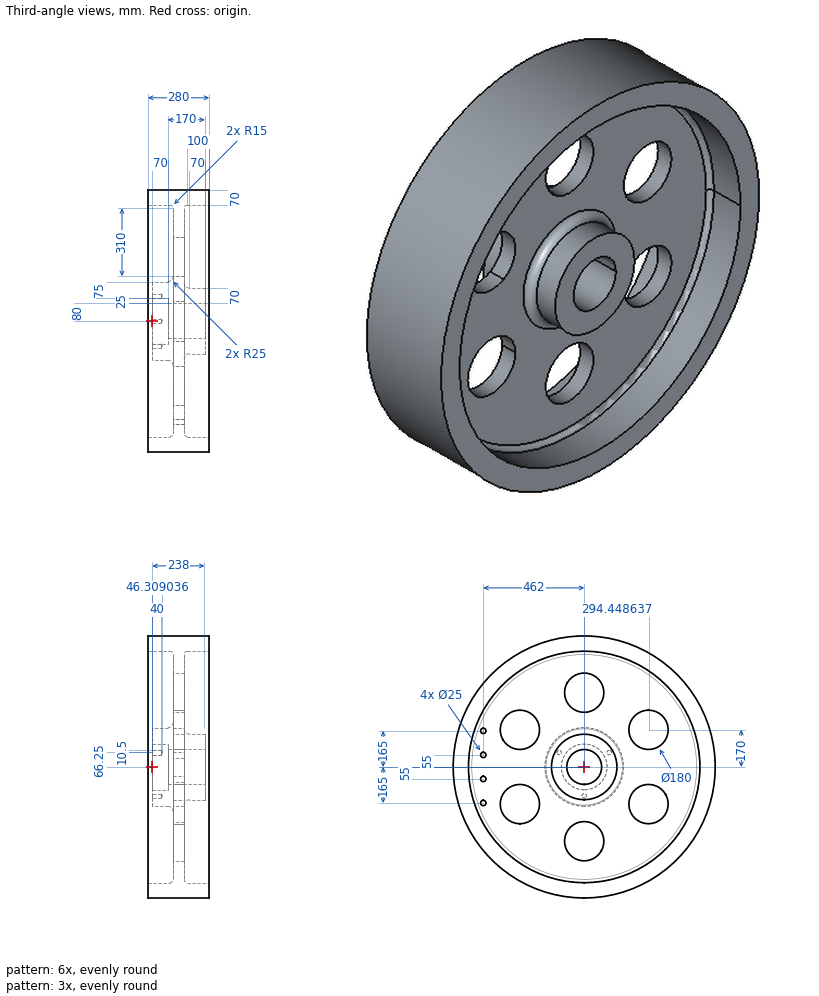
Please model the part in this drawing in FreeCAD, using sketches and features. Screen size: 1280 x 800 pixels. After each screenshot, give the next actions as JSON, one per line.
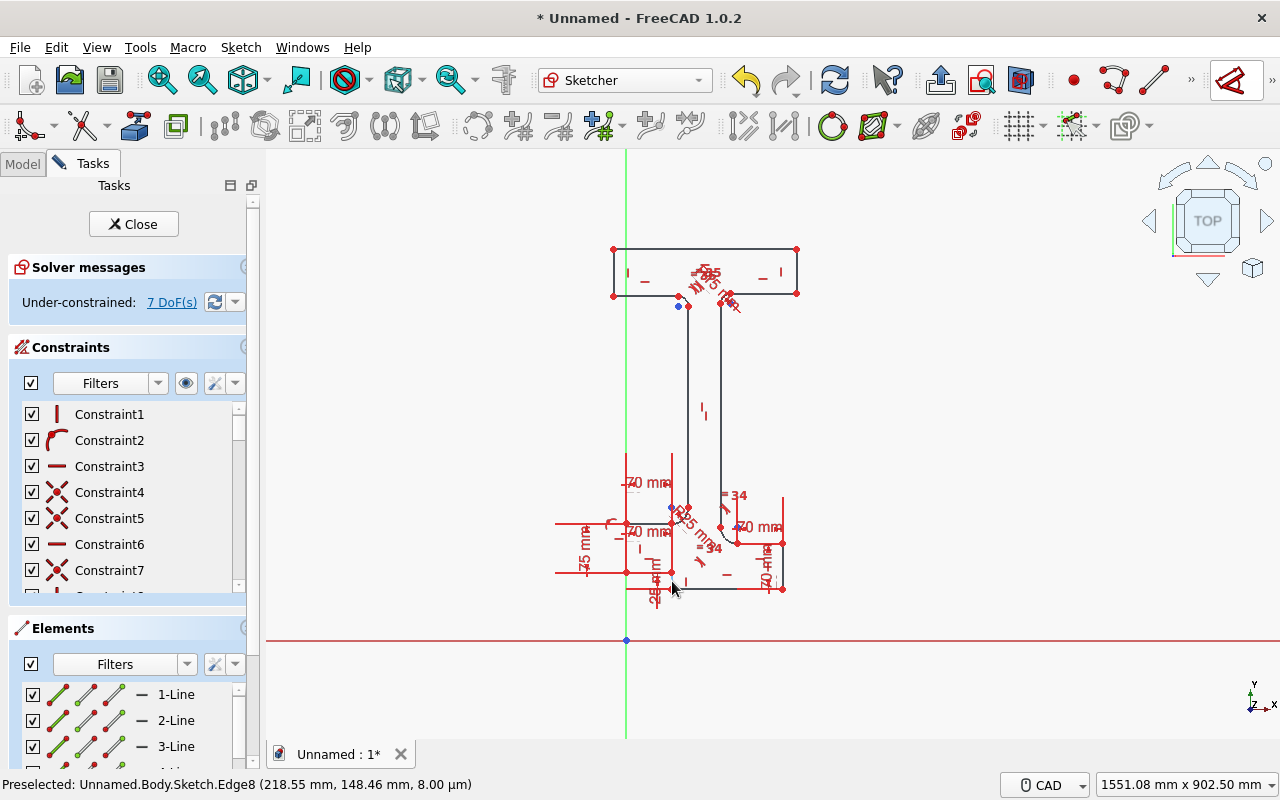
{"action": "left_click", "coordinate": [797, 280]}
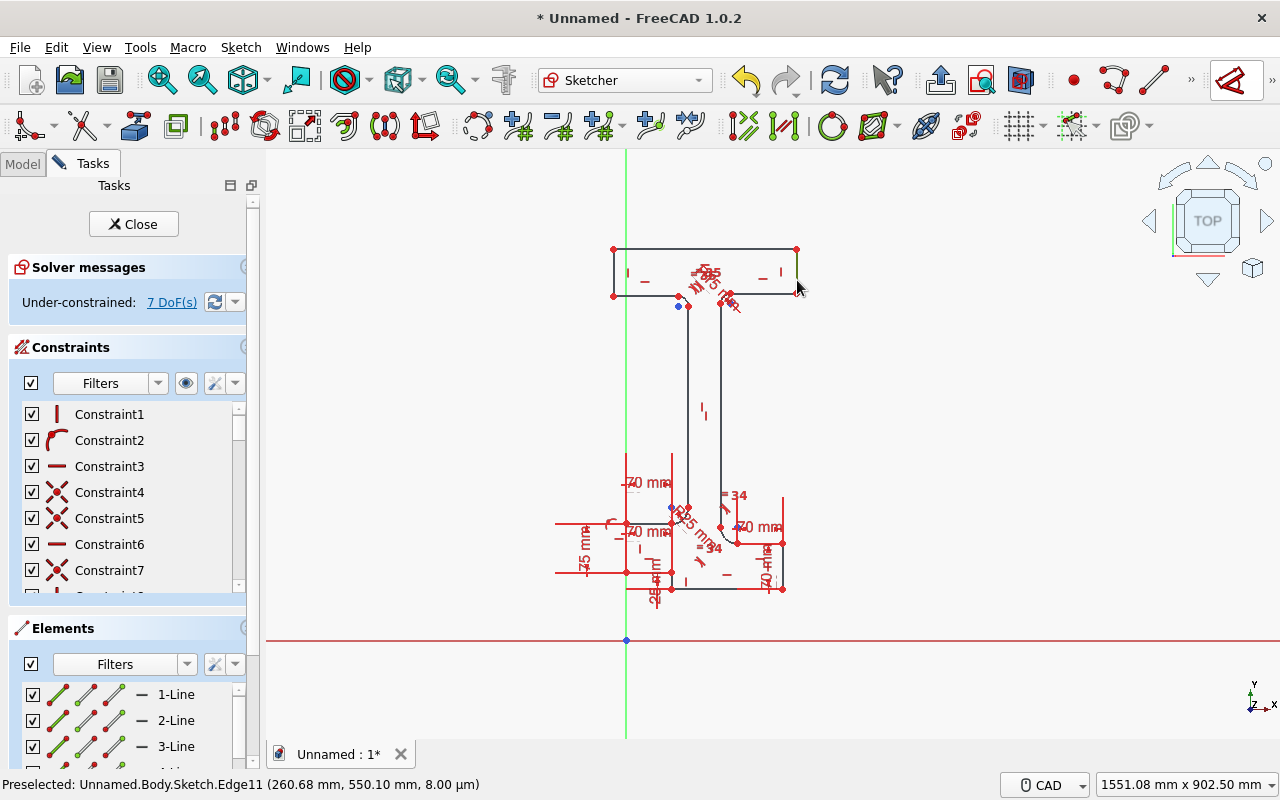
{"action": "left_click", "coordinate": [1258, 80]}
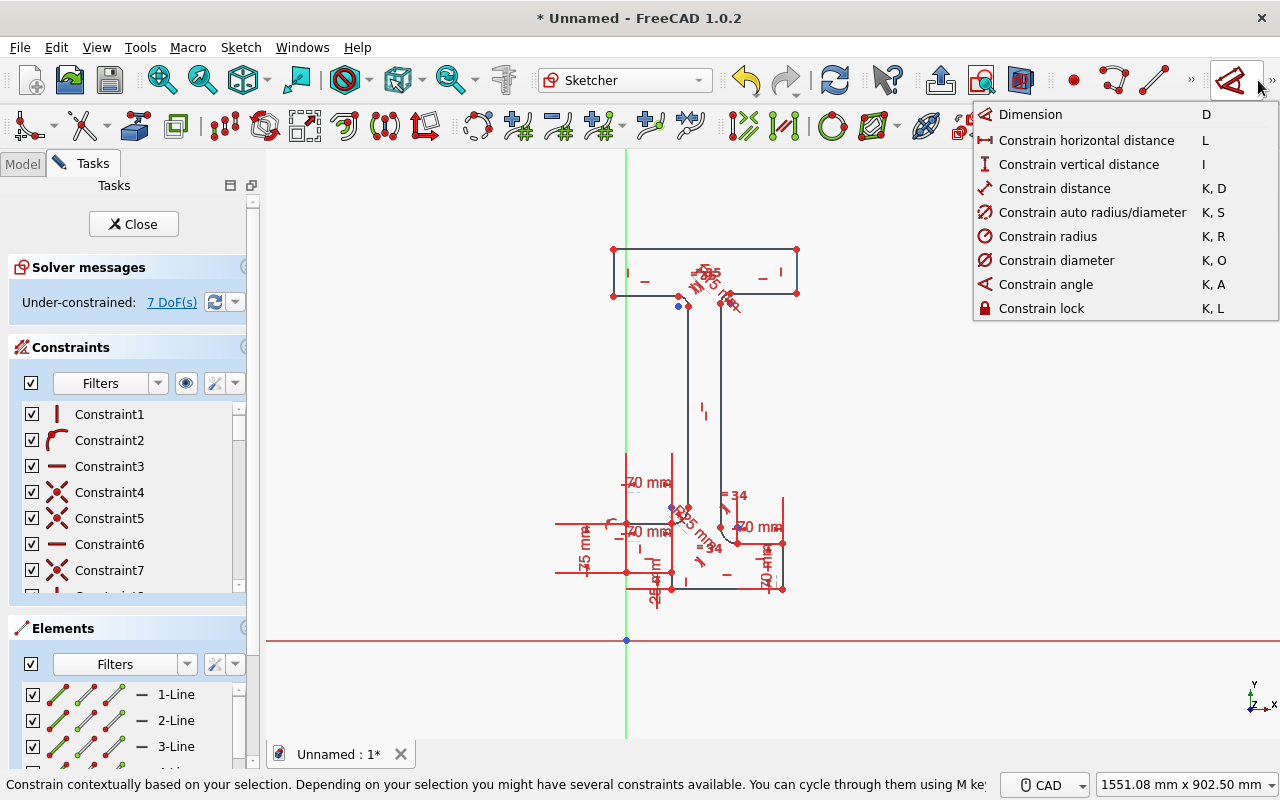
{"action": "left_click", "coordinate": [1126, 164]}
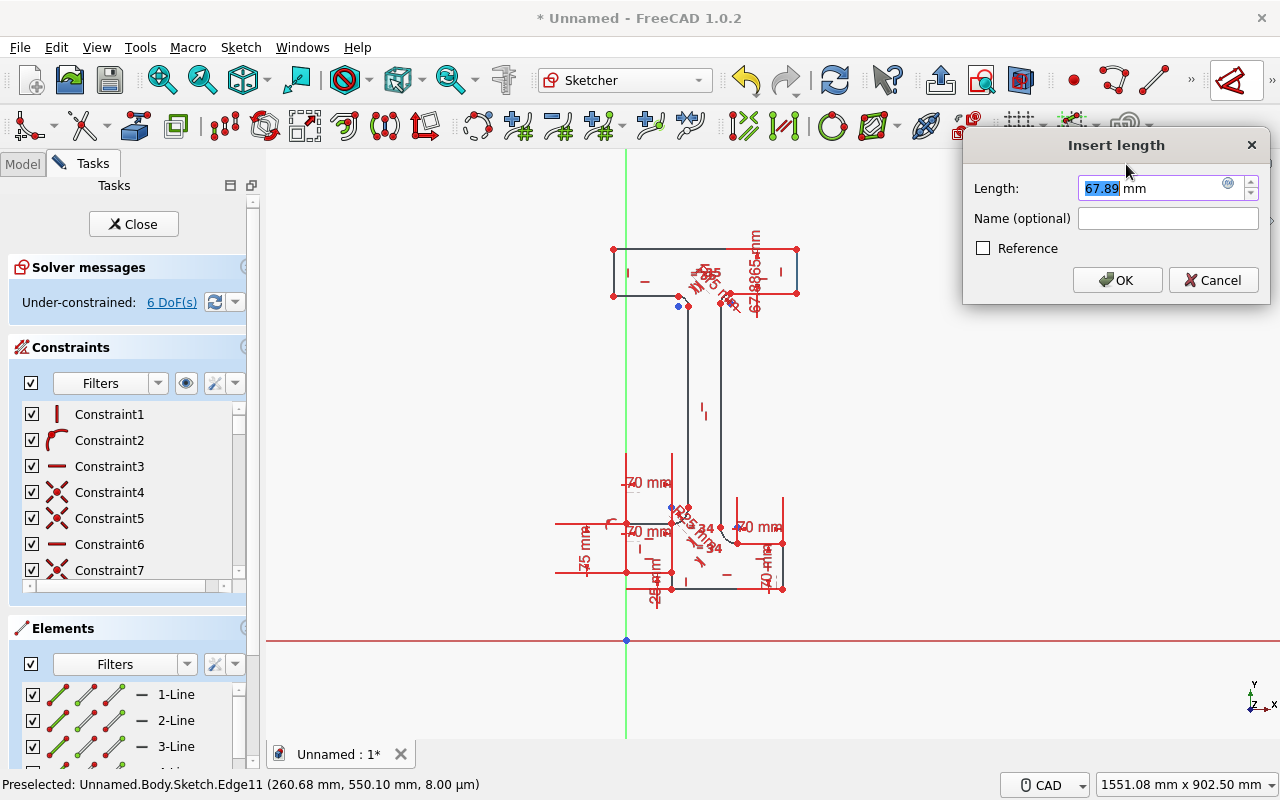
{"action": "type", "text": "70"}
{"action": "key", "text": "Return"}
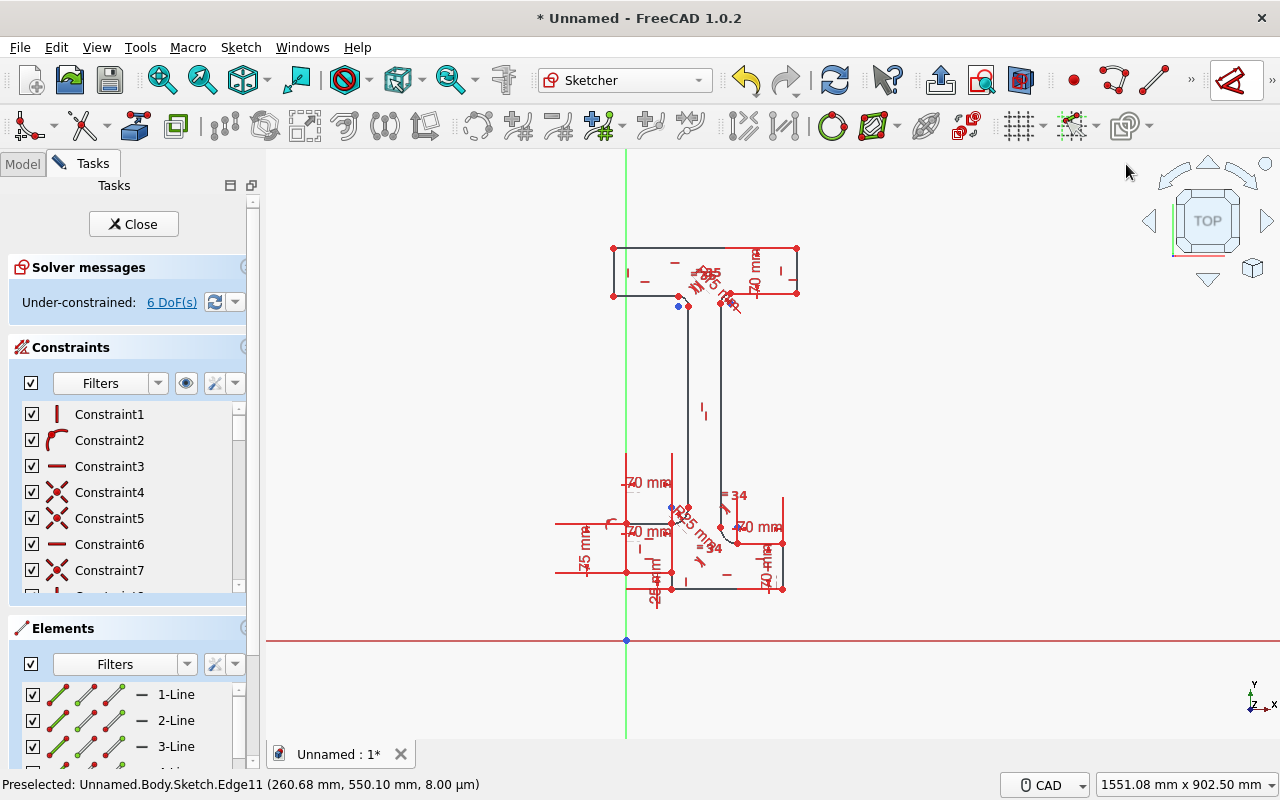
{"action": "left_click", "coordinate": [614, 262]}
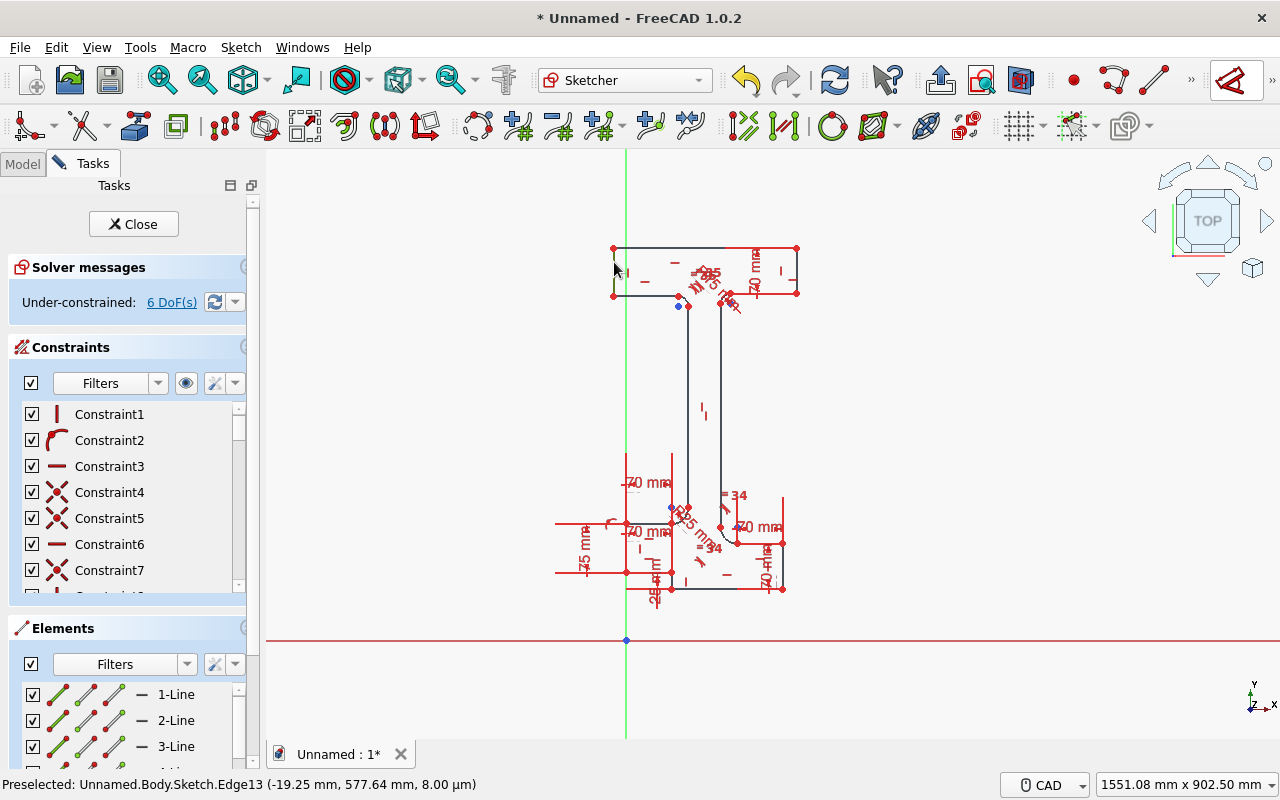
{"action": "key", "text": "i"}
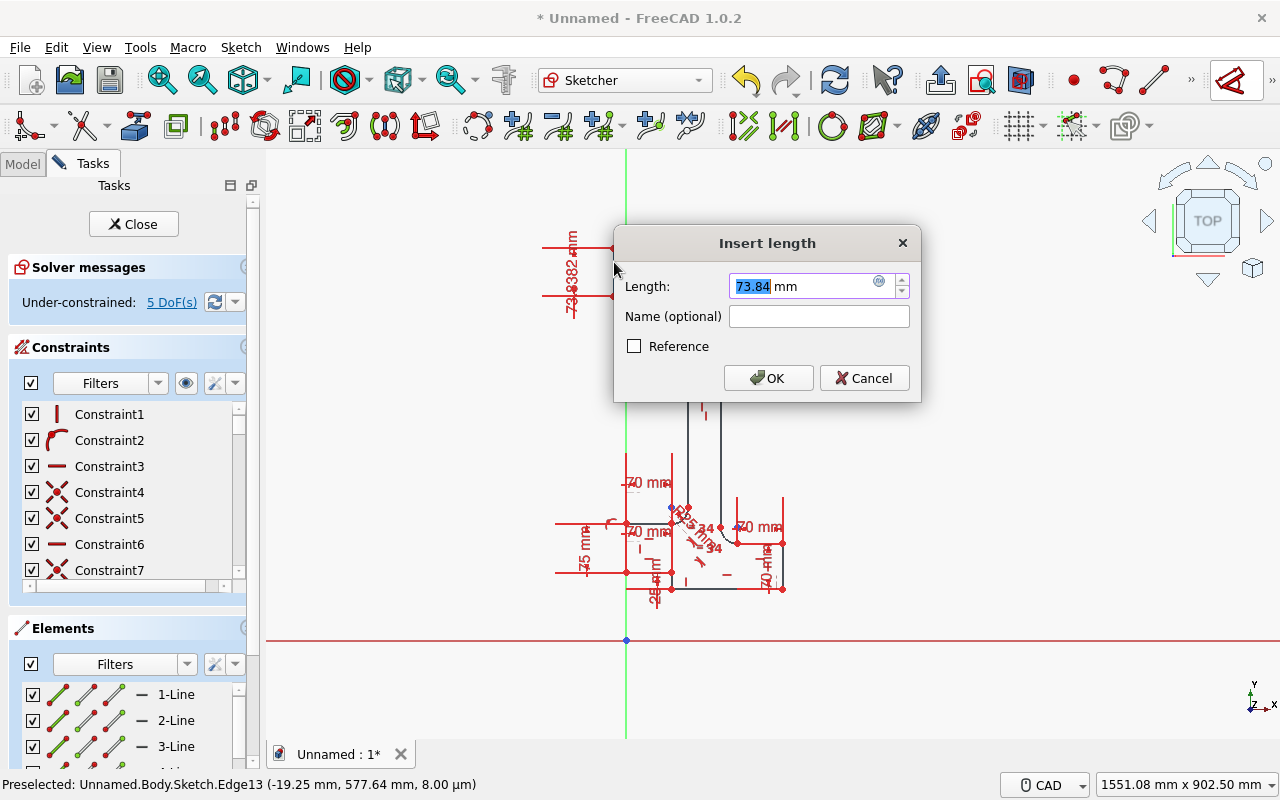
{"action": "type", "text": "70"}
{"action": "key", "text": "Return"}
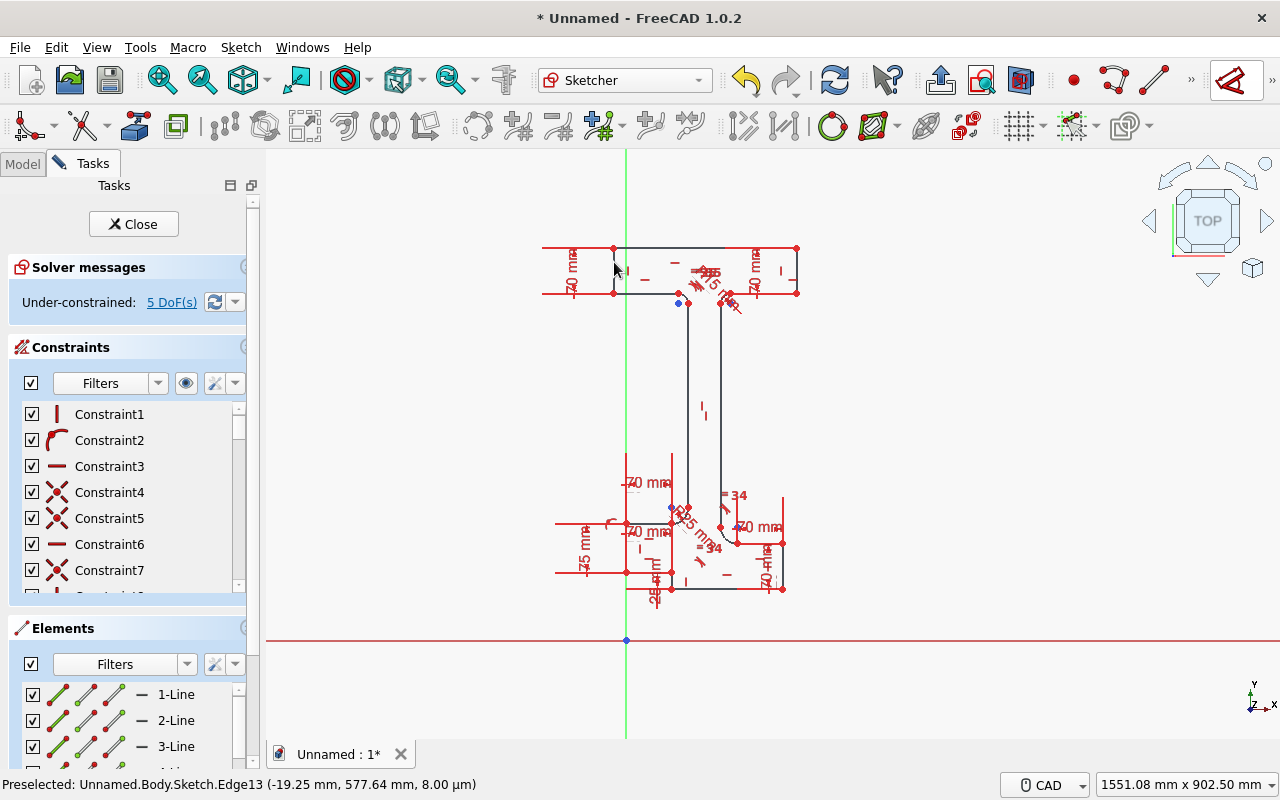
{"action": "left_click", "coordinate": [688, 365]}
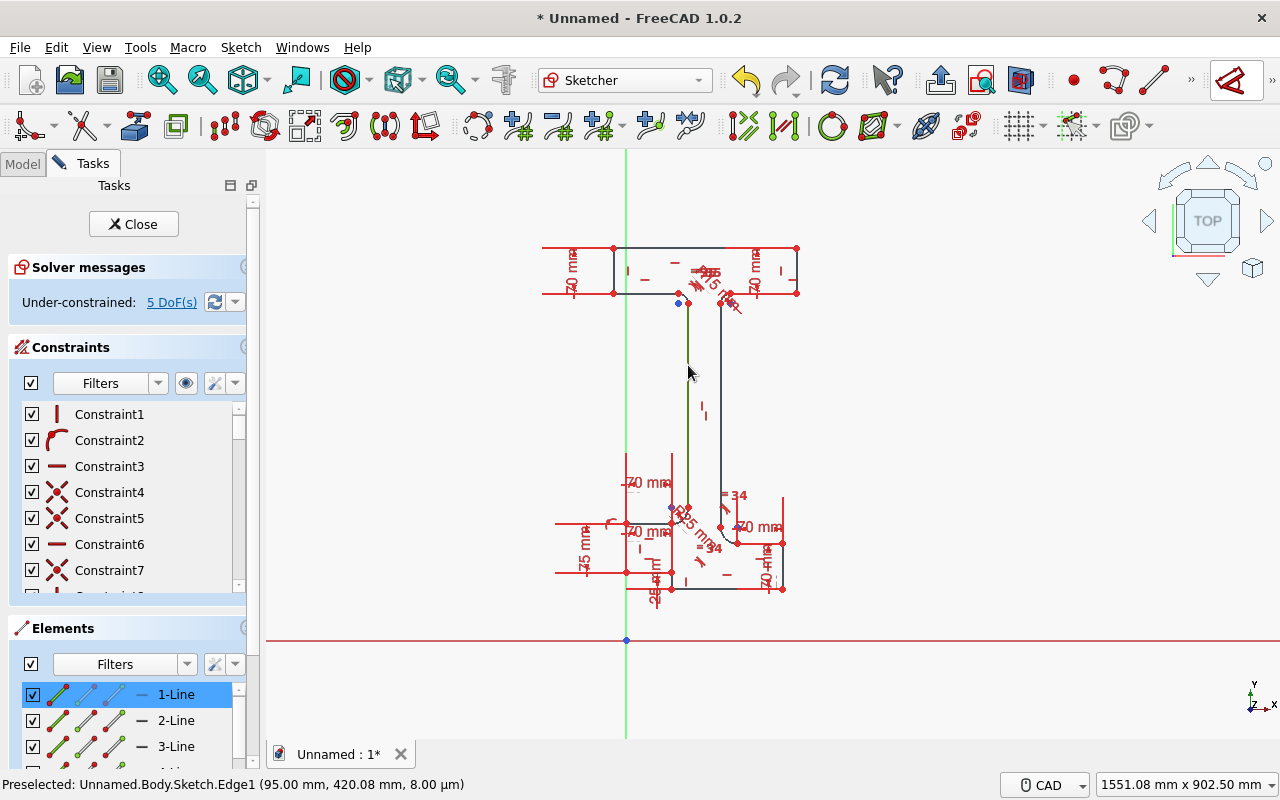
{"action": "left_click", "coordinate": [1258, 80]}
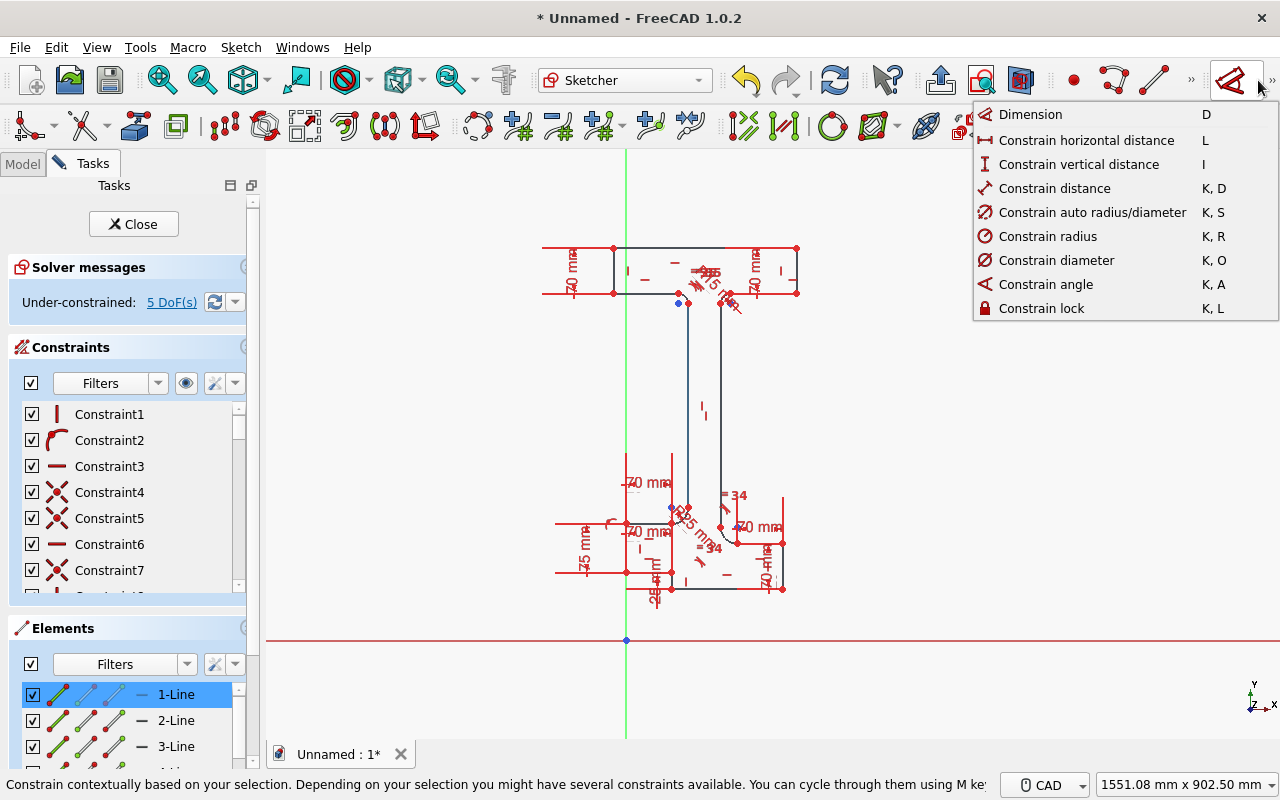
{"action": "left_click", "coordinate": [1126, 164]}